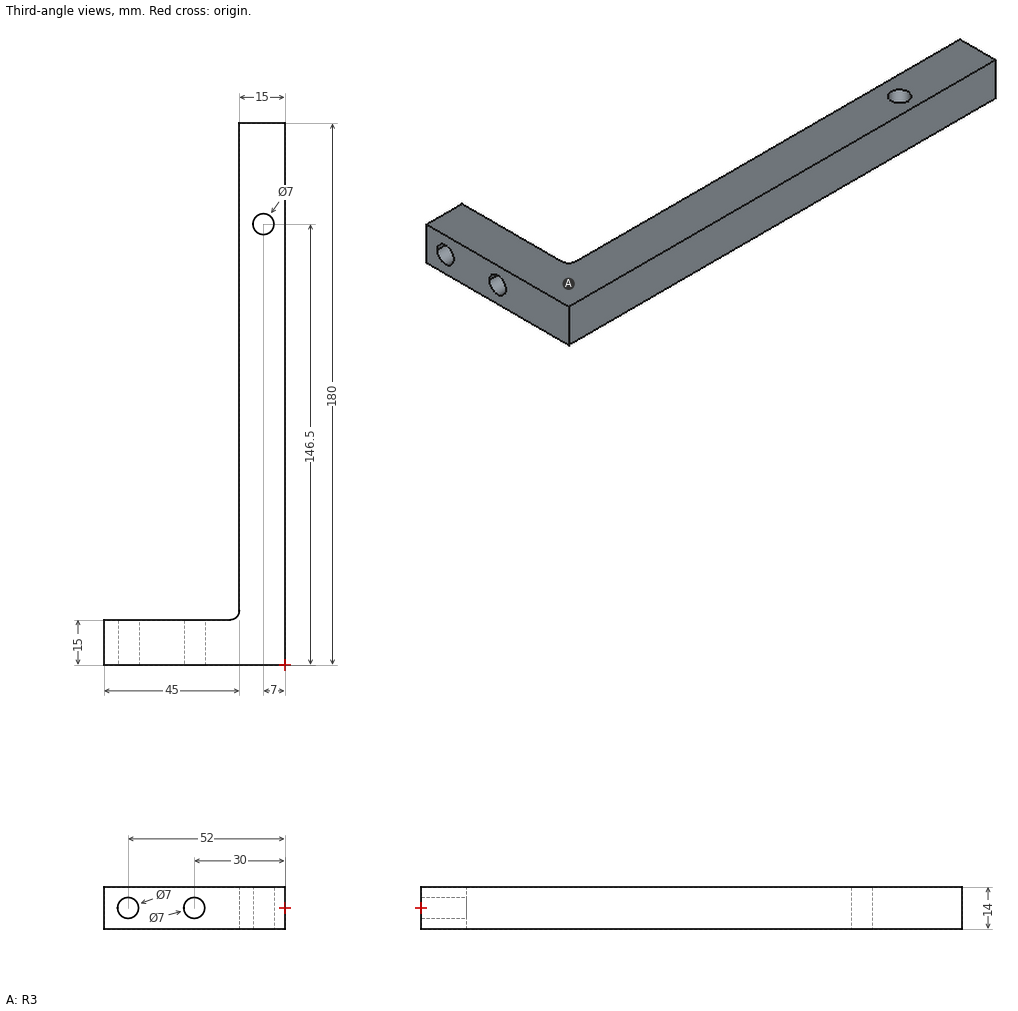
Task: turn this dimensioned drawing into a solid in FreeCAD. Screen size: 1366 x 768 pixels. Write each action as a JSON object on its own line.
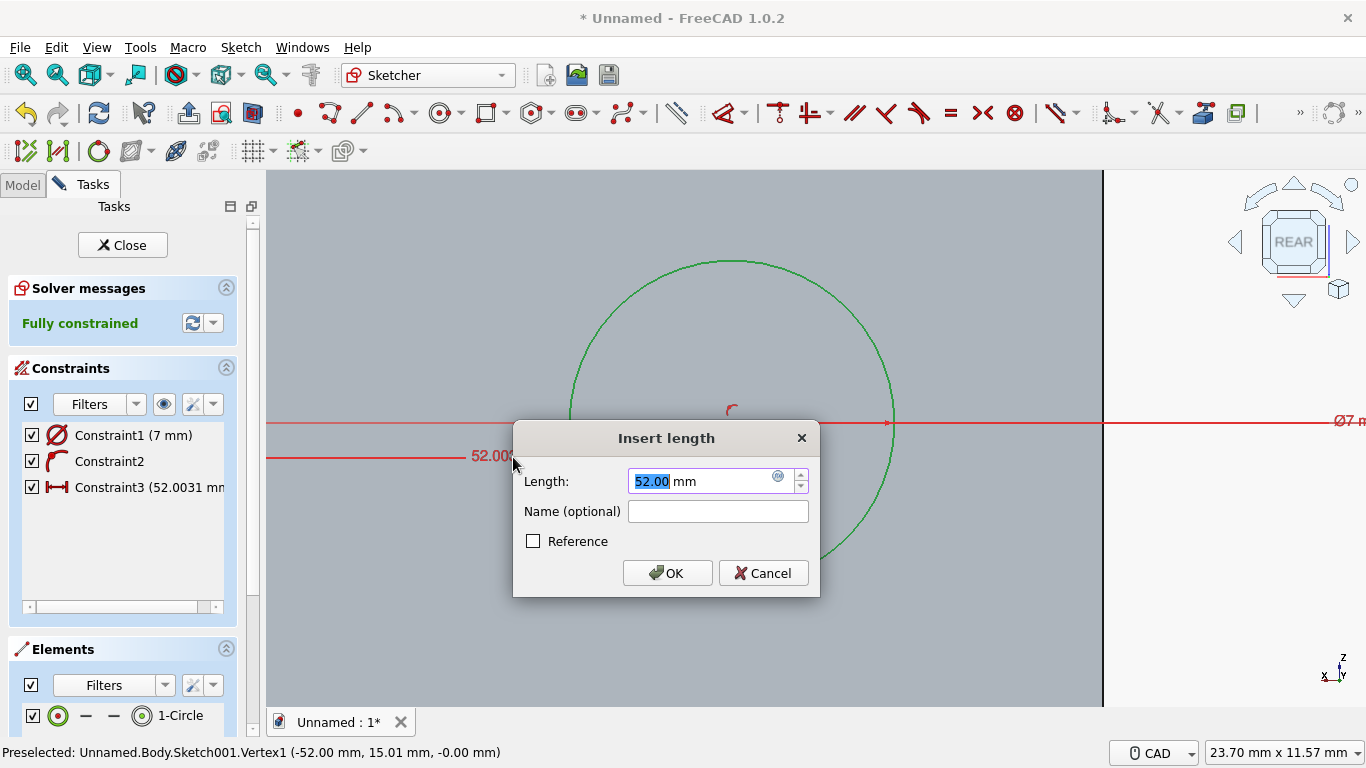
{"action": "type", "text": "52"}
{"action": "key", "text": "Return"}
{"action": "key", "text": "Escape"}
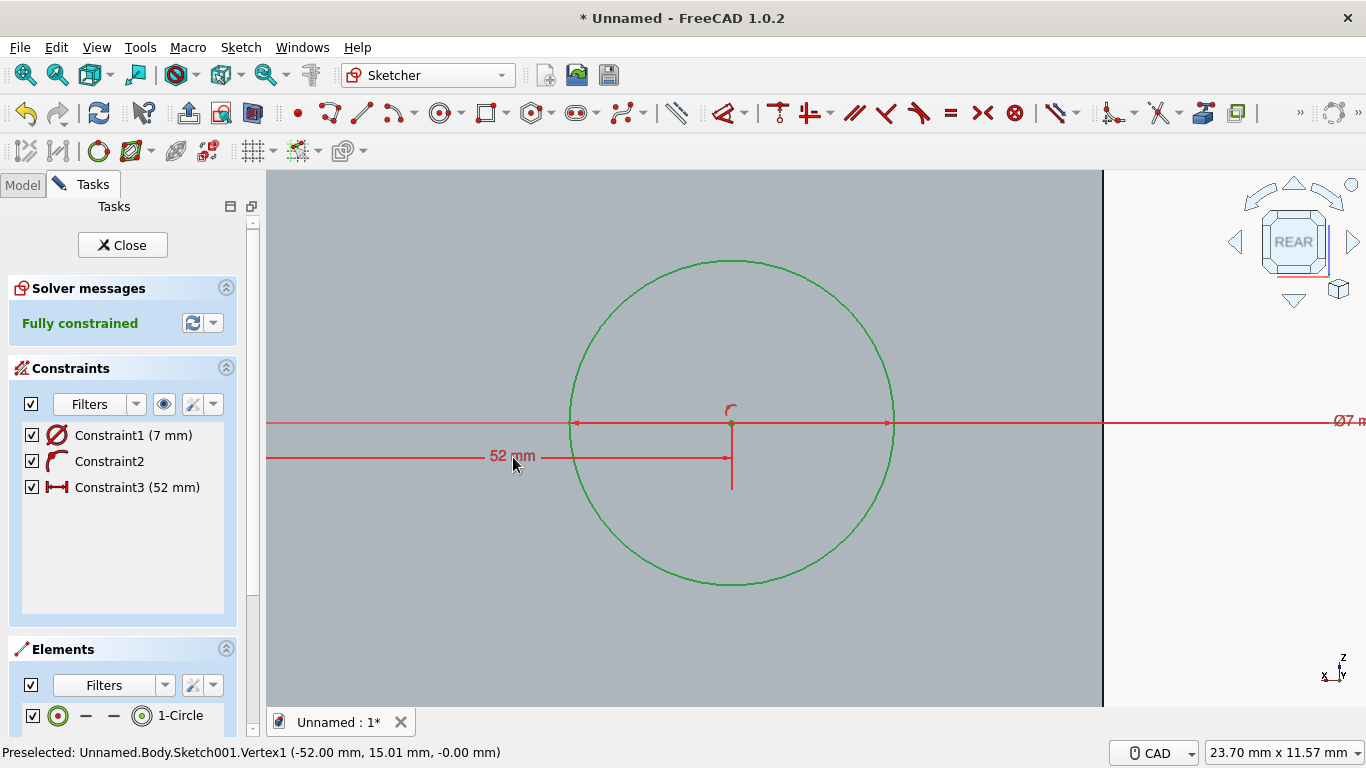
{"action": "left_click", "coordinate": [123, 245]}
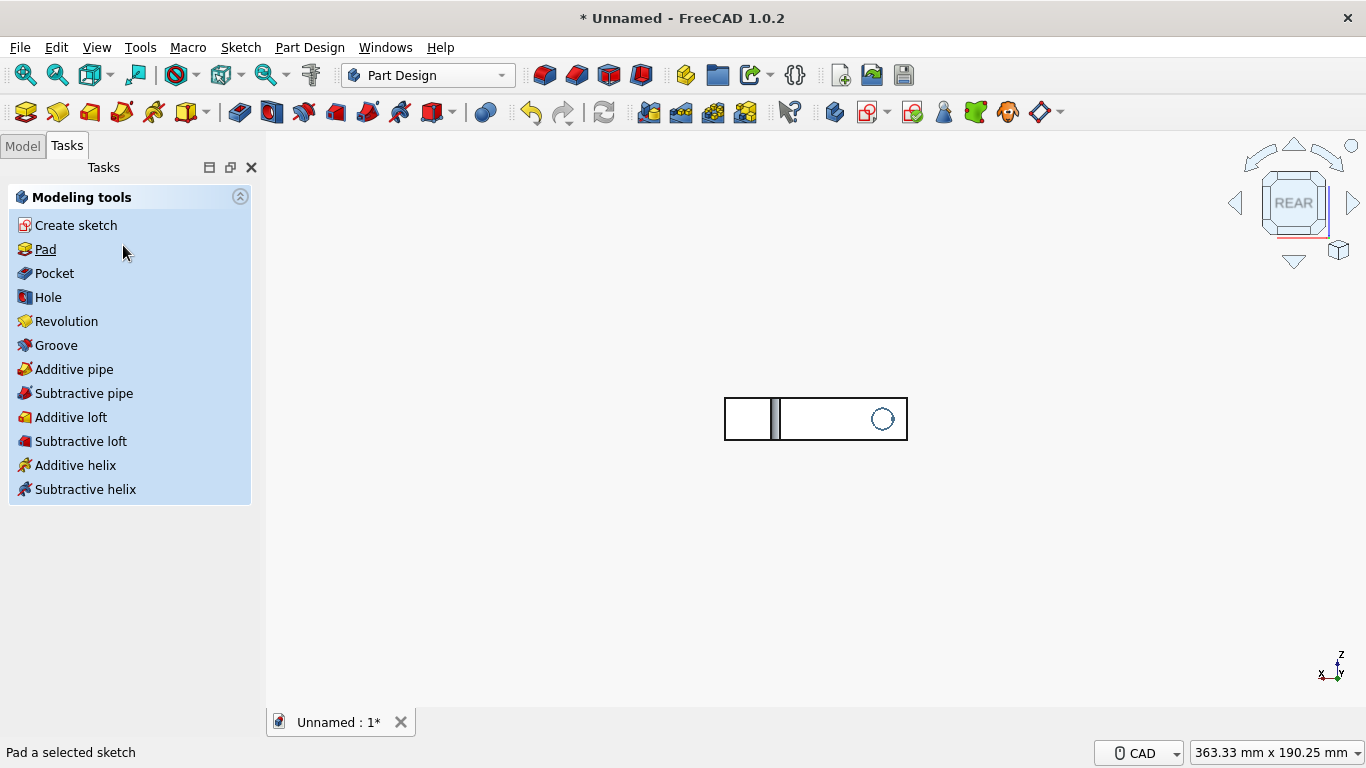
{"action": "left_click", "coordinate": [240, 112]}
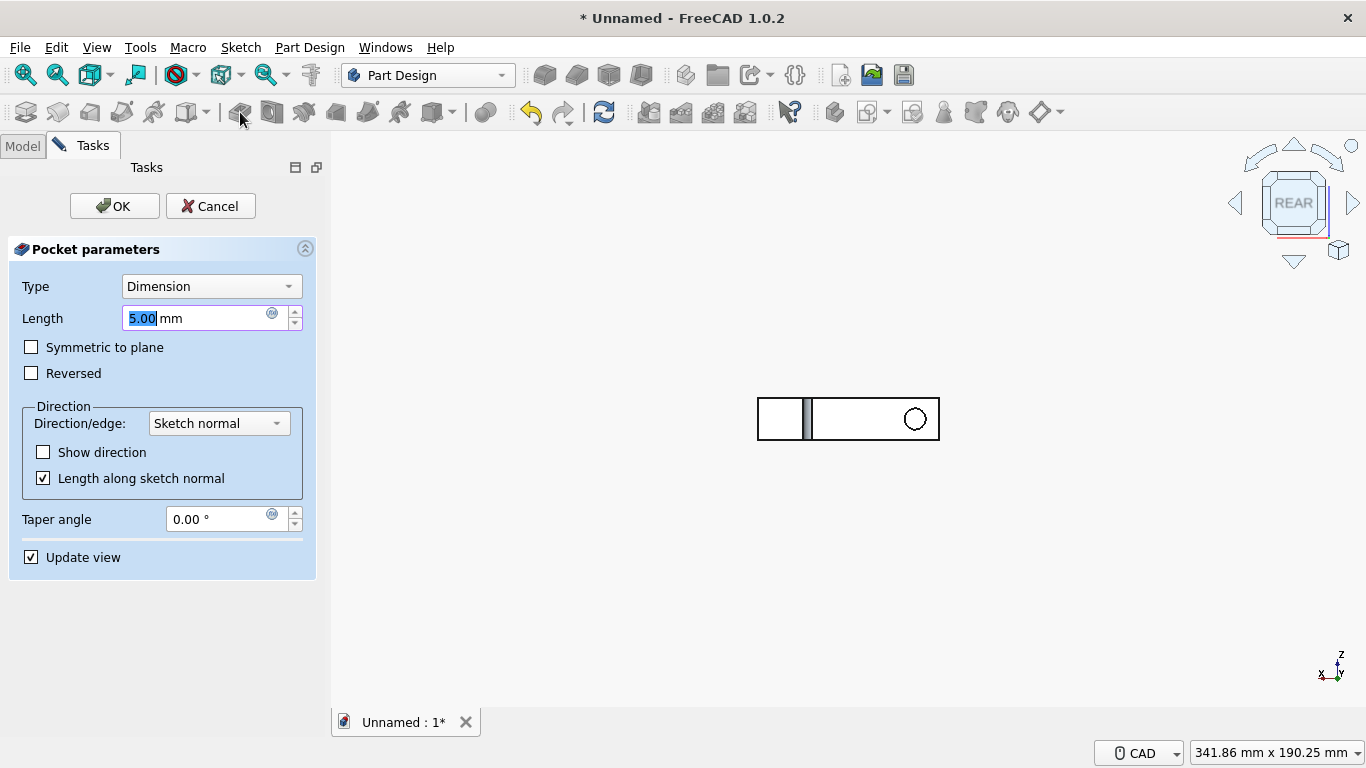
{"action": "left_click", "coordinate": [212, 286]}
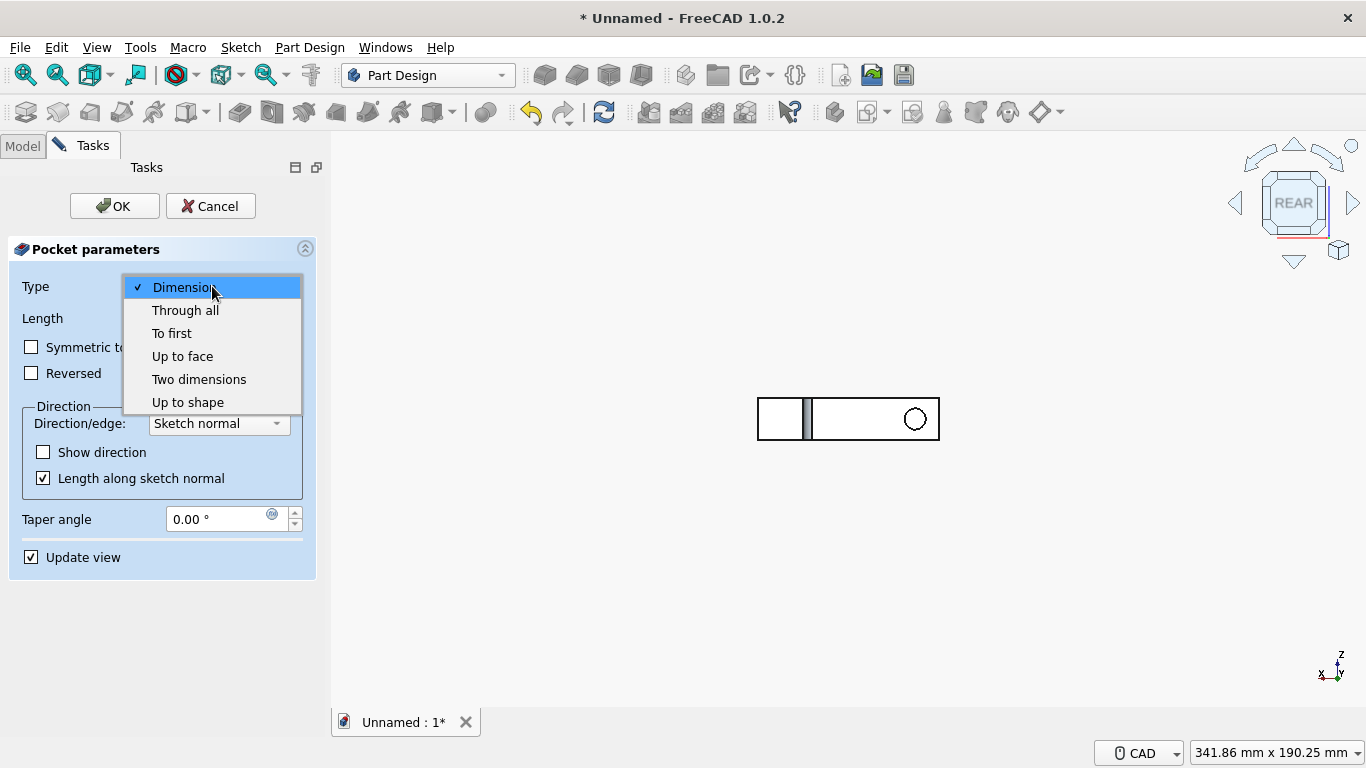
{"action": "left_click", "coordinate": [212, 334]}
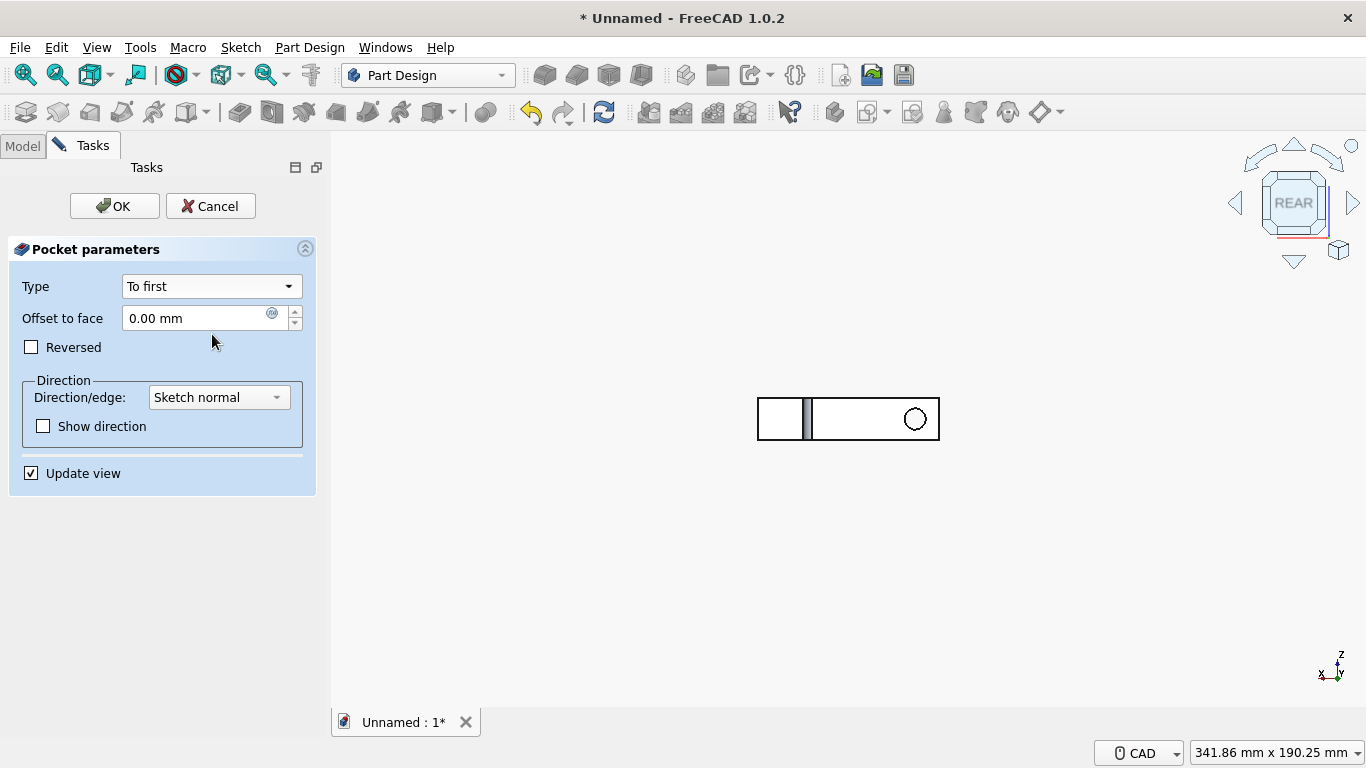
{"action": "left_click", "coordinate": [115, 206]}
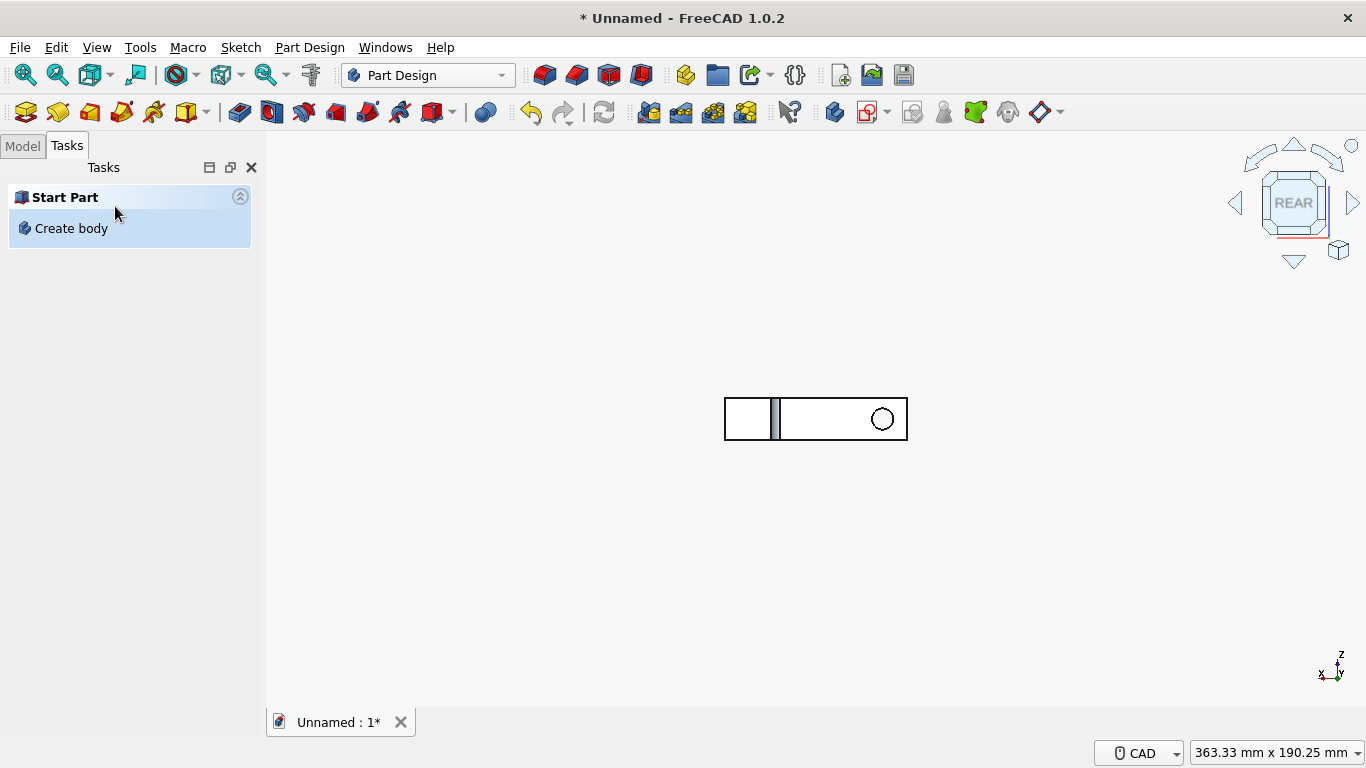
{"action": "left_click", "coordinate": [26, 76]}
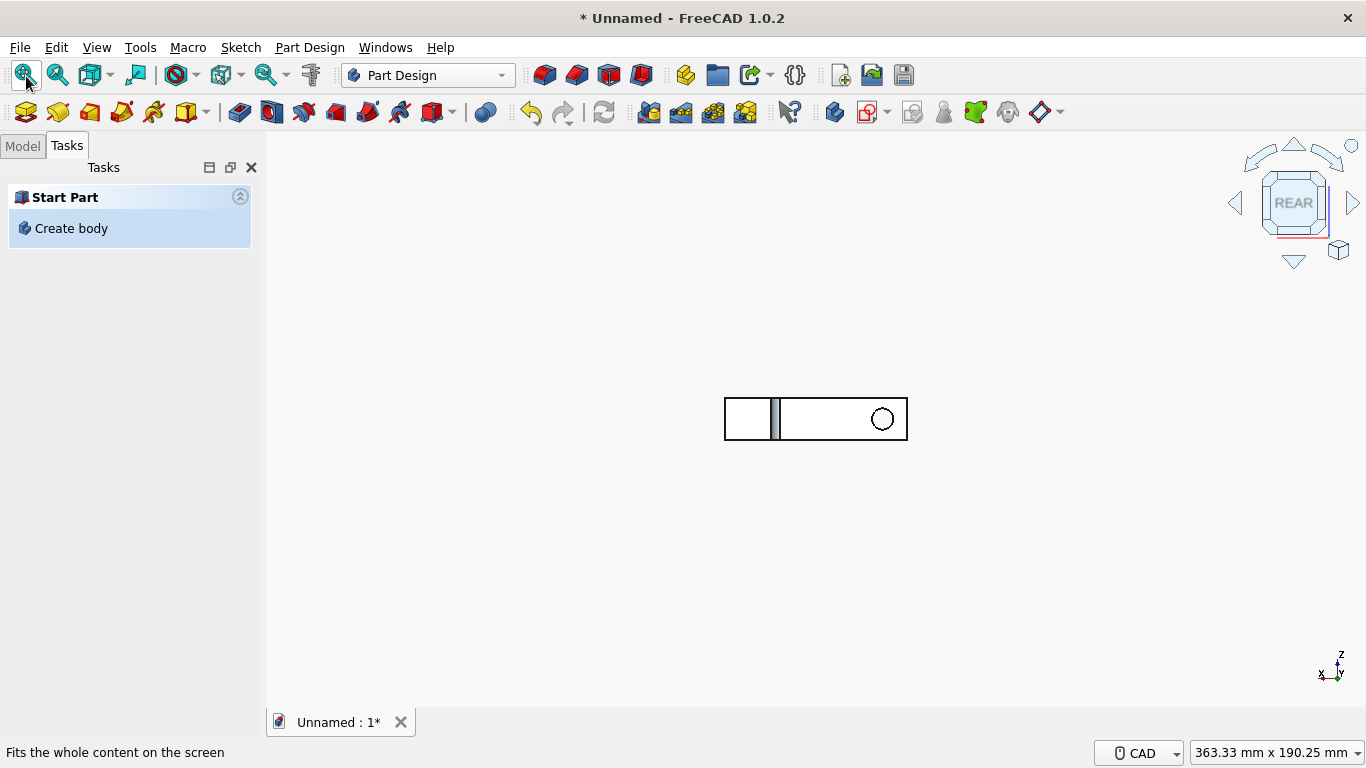
{"action": "left_click", "coordinate": [807, 418]}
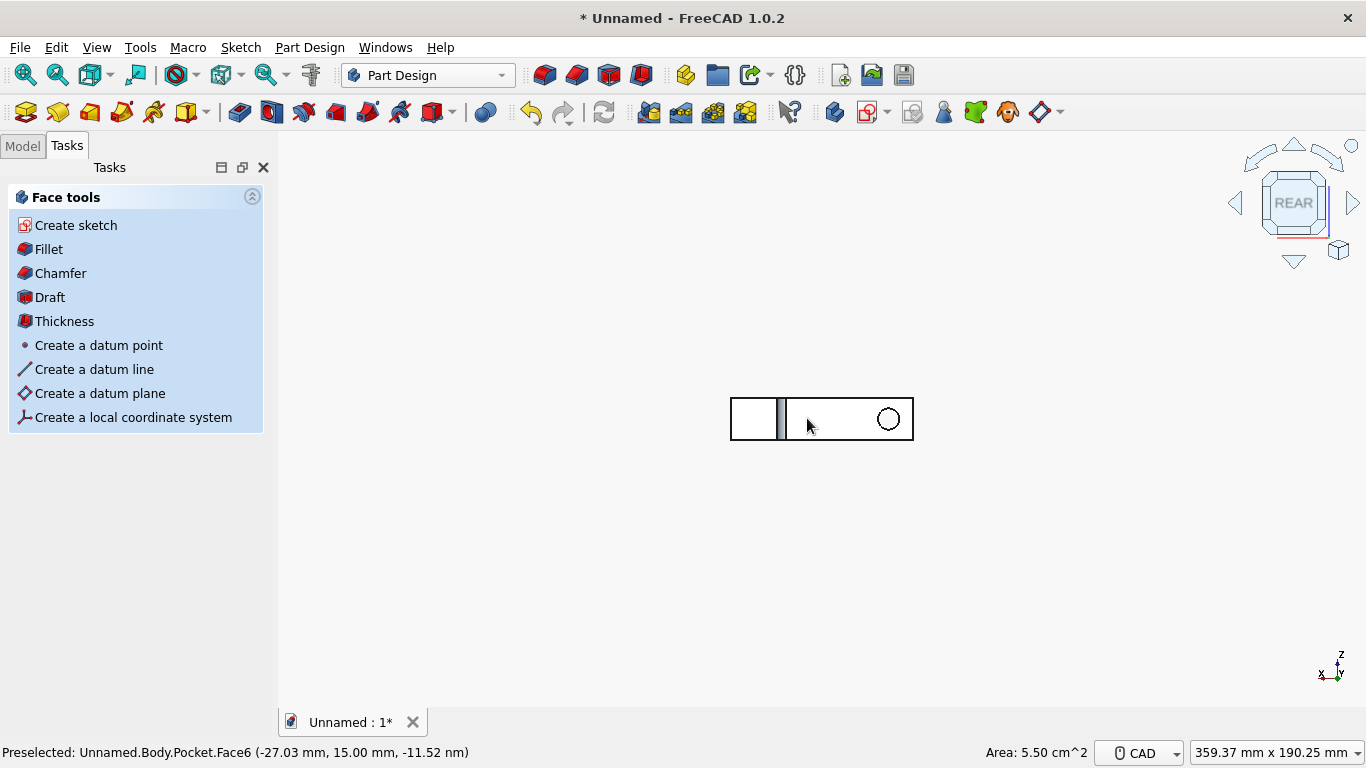
{"action": "left_click", "coordinate": [868, 112]}